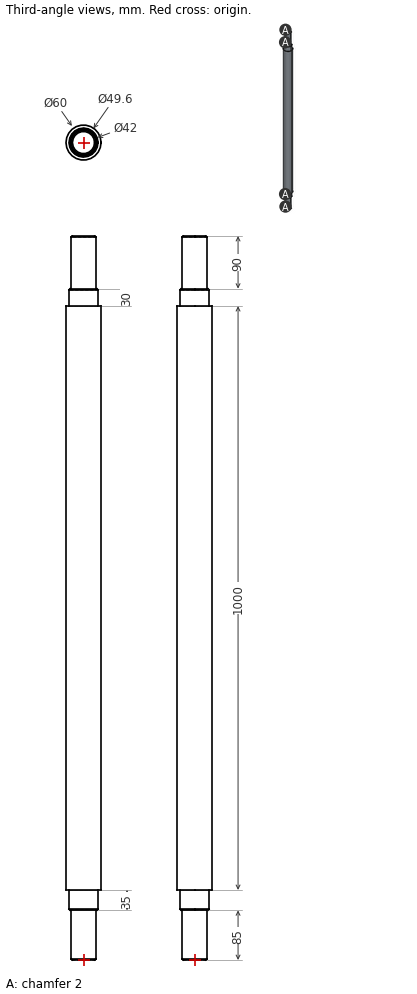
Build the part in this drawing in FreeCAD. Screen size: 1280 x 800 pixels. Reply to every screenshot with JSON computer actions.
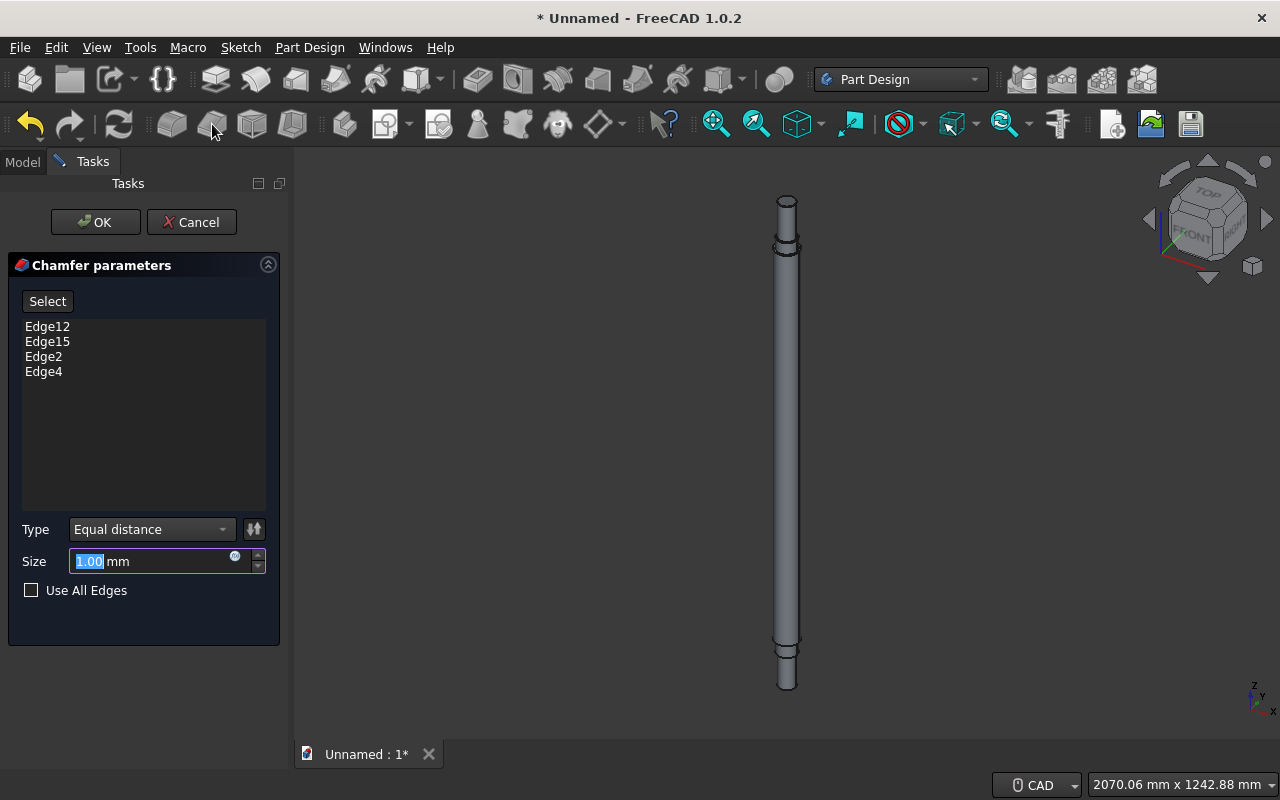
{"action": "type", "text": "2"}
{"action": "key", "text": "Tab"}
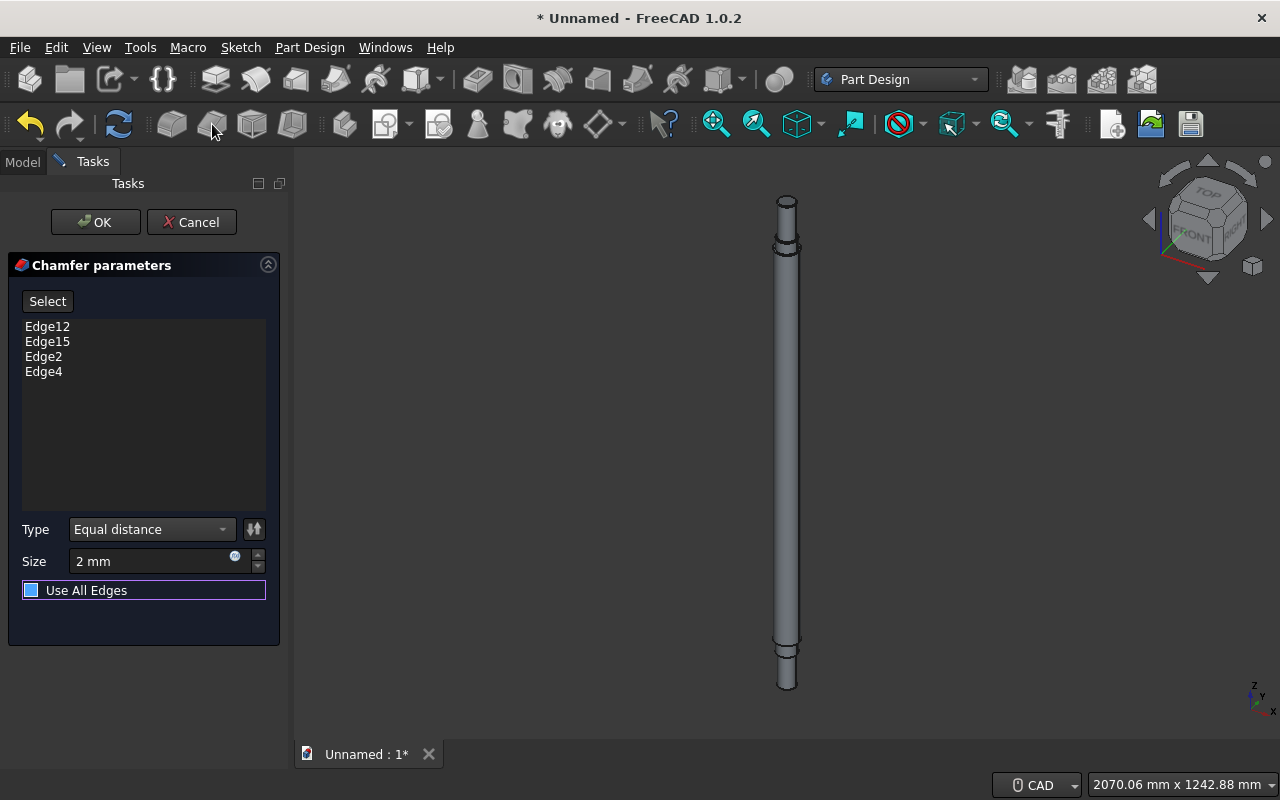
{"action": "left_click", "coordinate": [96, 222]}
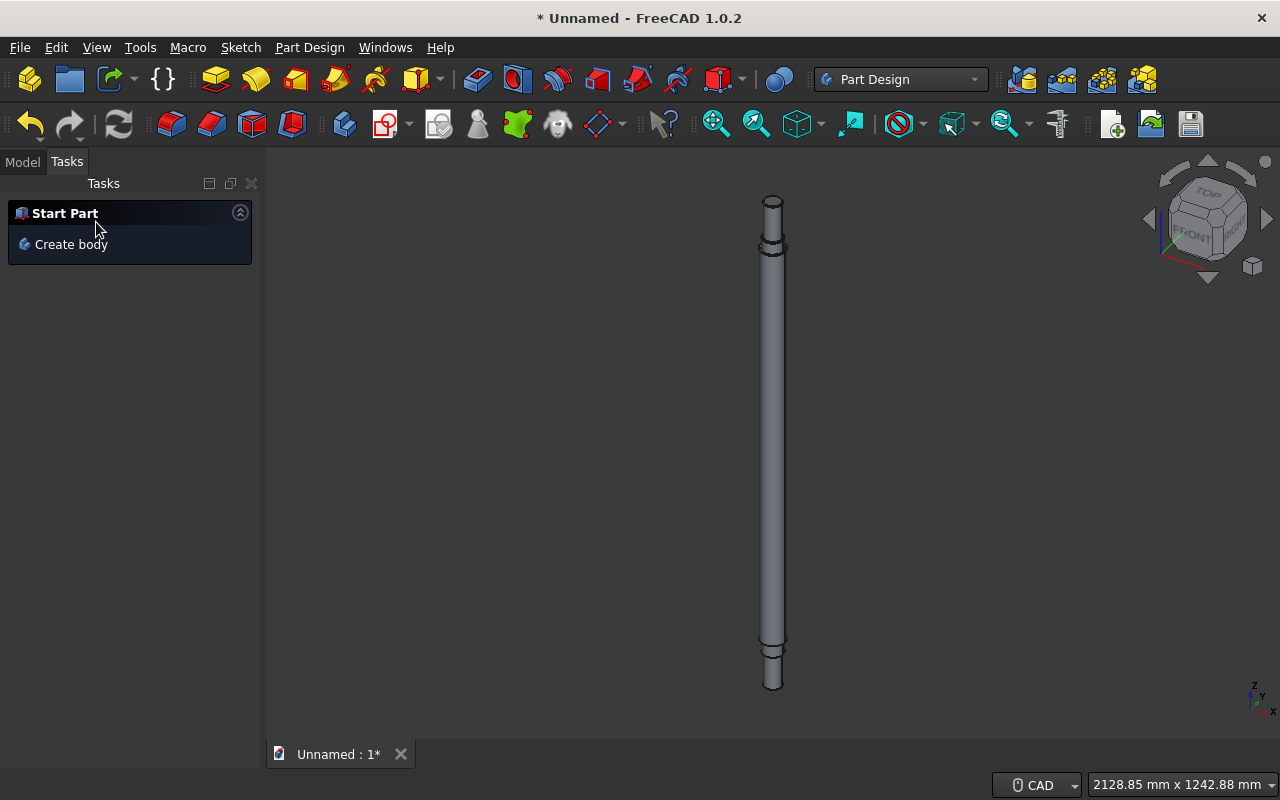
{"action": "key", "text": "0"}